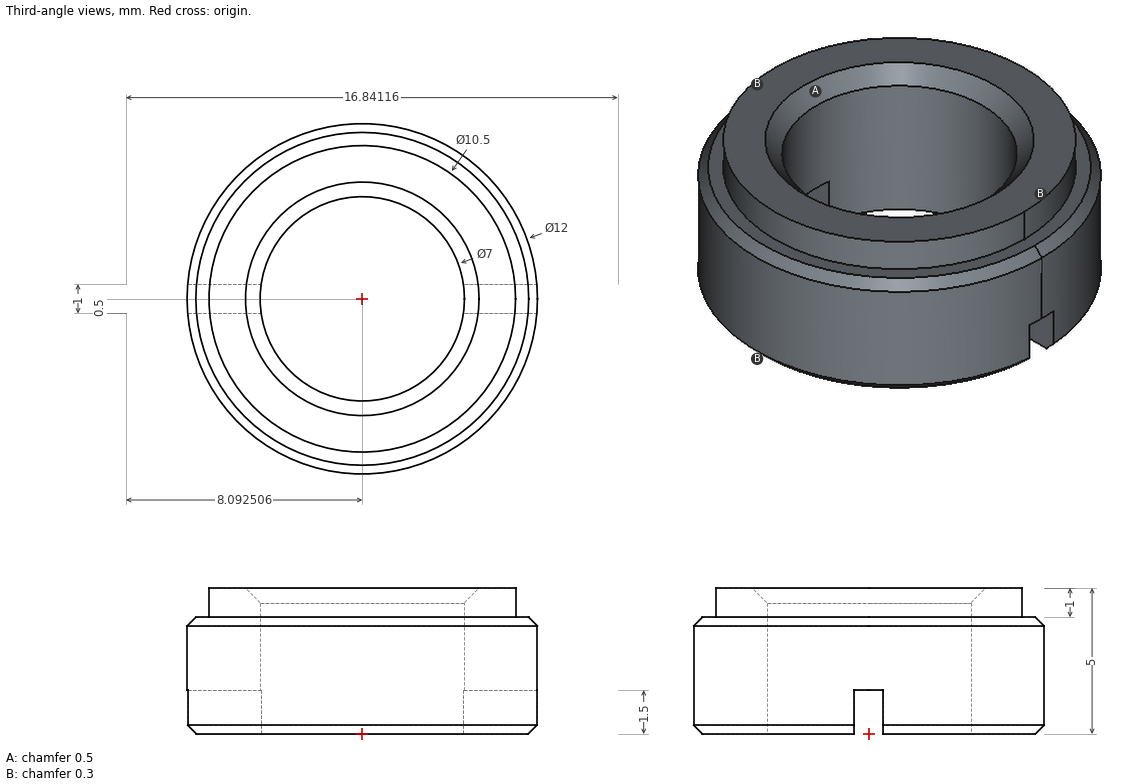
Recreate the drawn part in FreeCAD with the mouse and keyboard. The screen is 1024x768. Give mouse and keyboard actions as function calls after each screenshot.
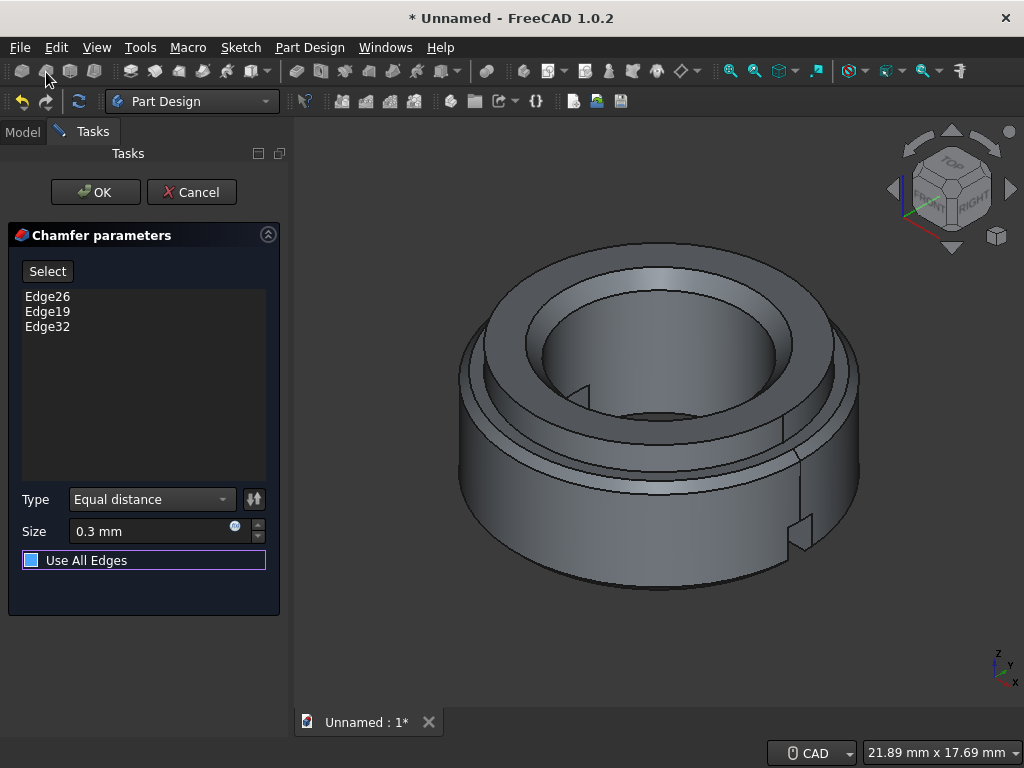
click(96, 192)